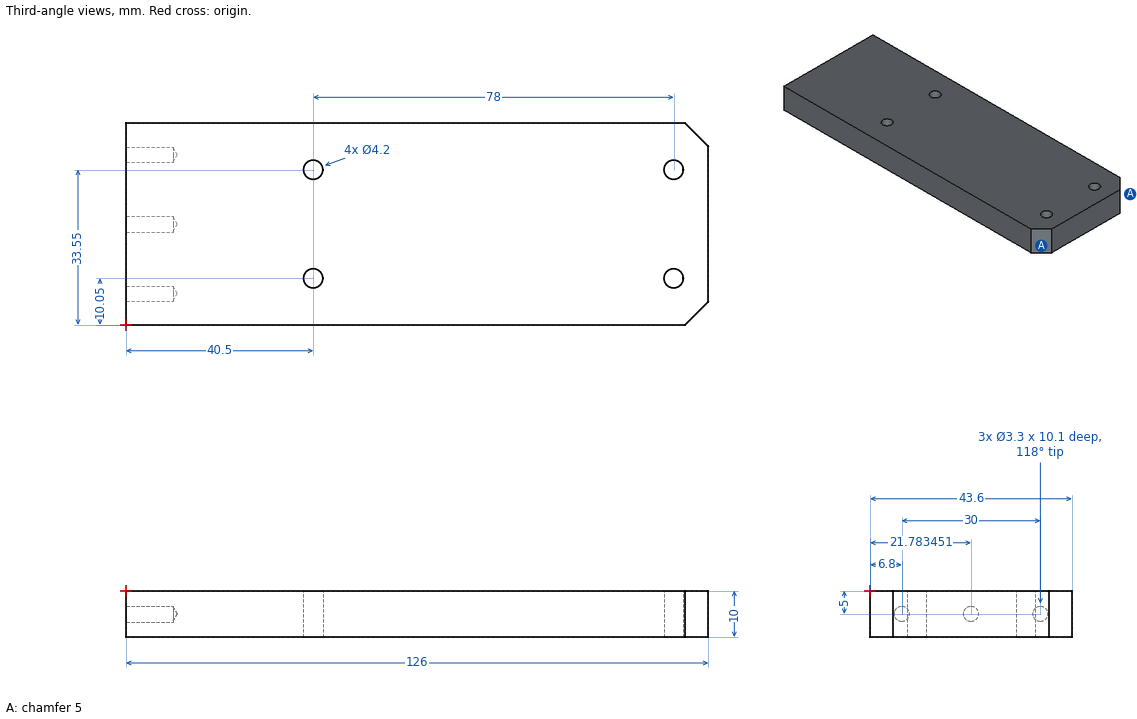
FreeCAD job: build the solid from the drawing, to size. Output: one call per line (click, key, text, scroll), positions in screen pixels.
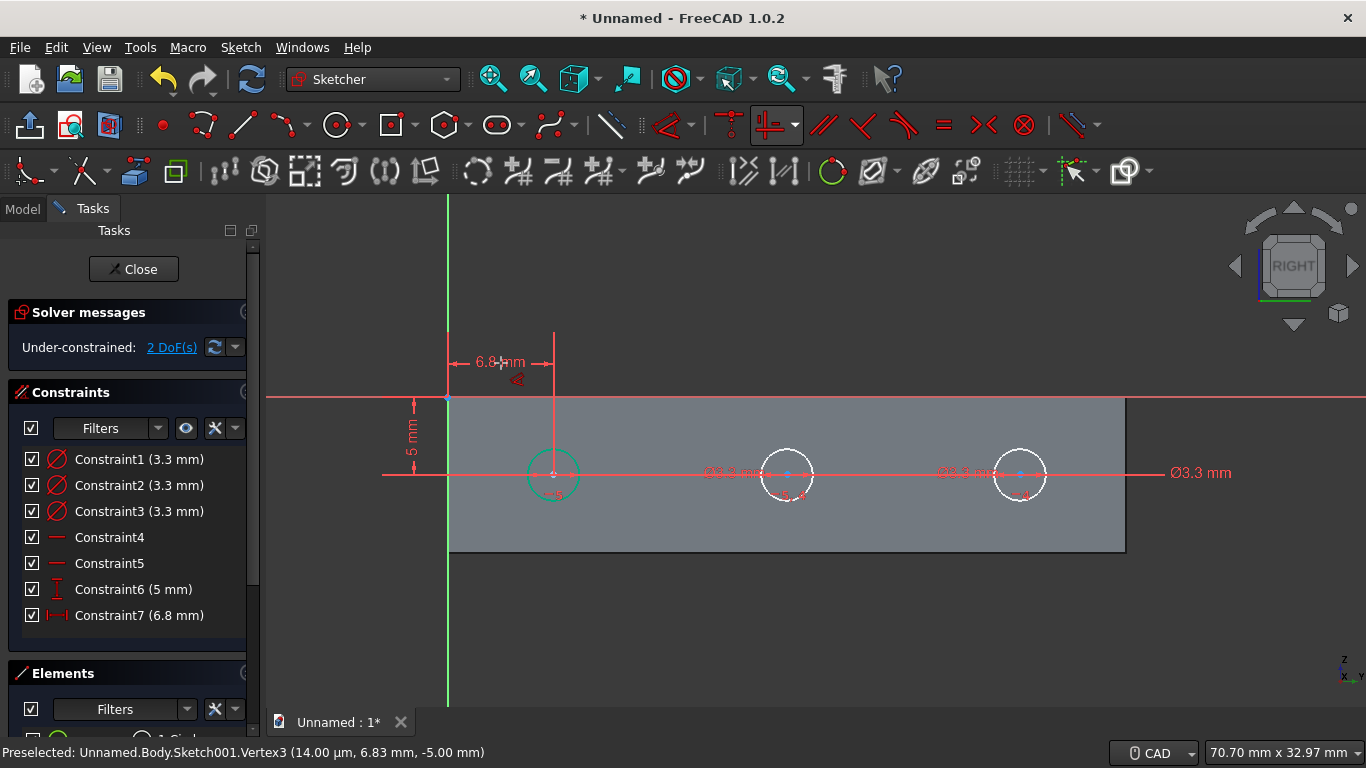
click(1020, 475)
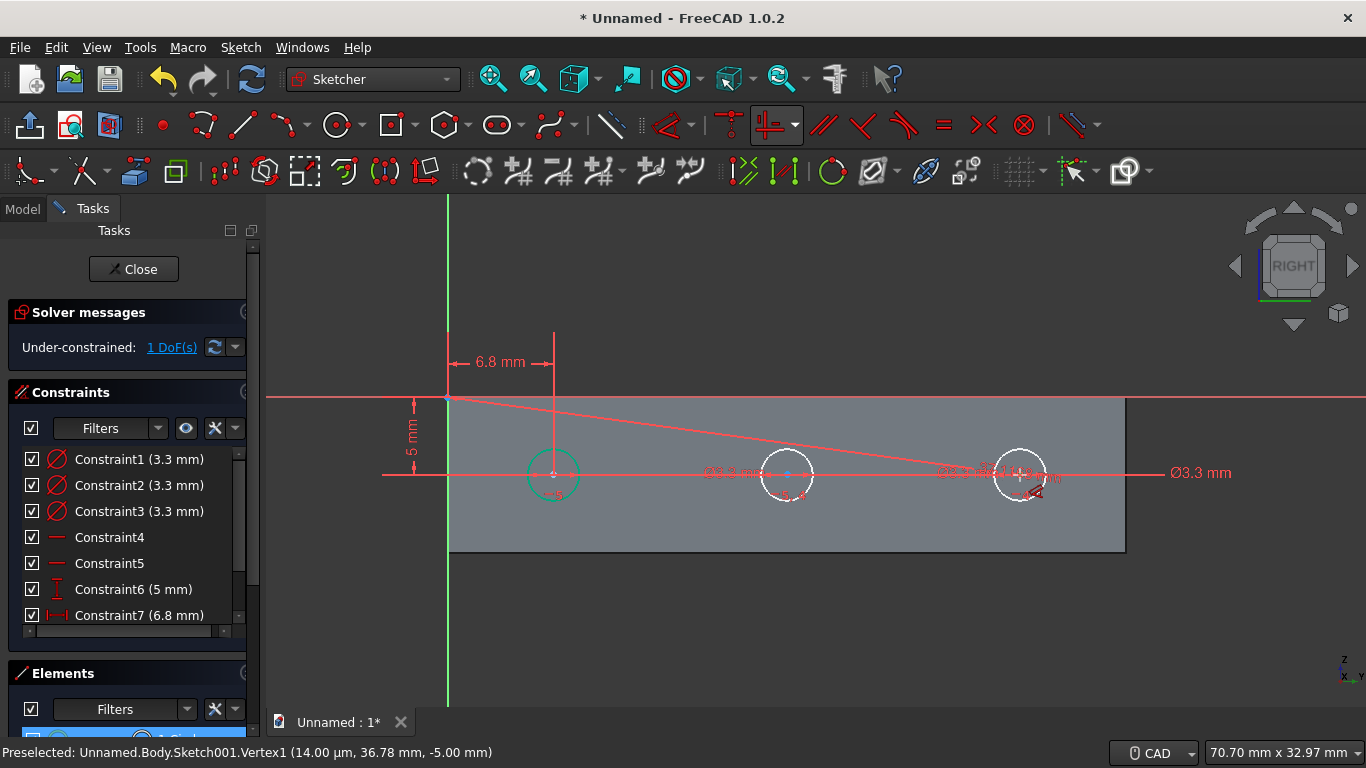
click(554, 475)
click(680, 509)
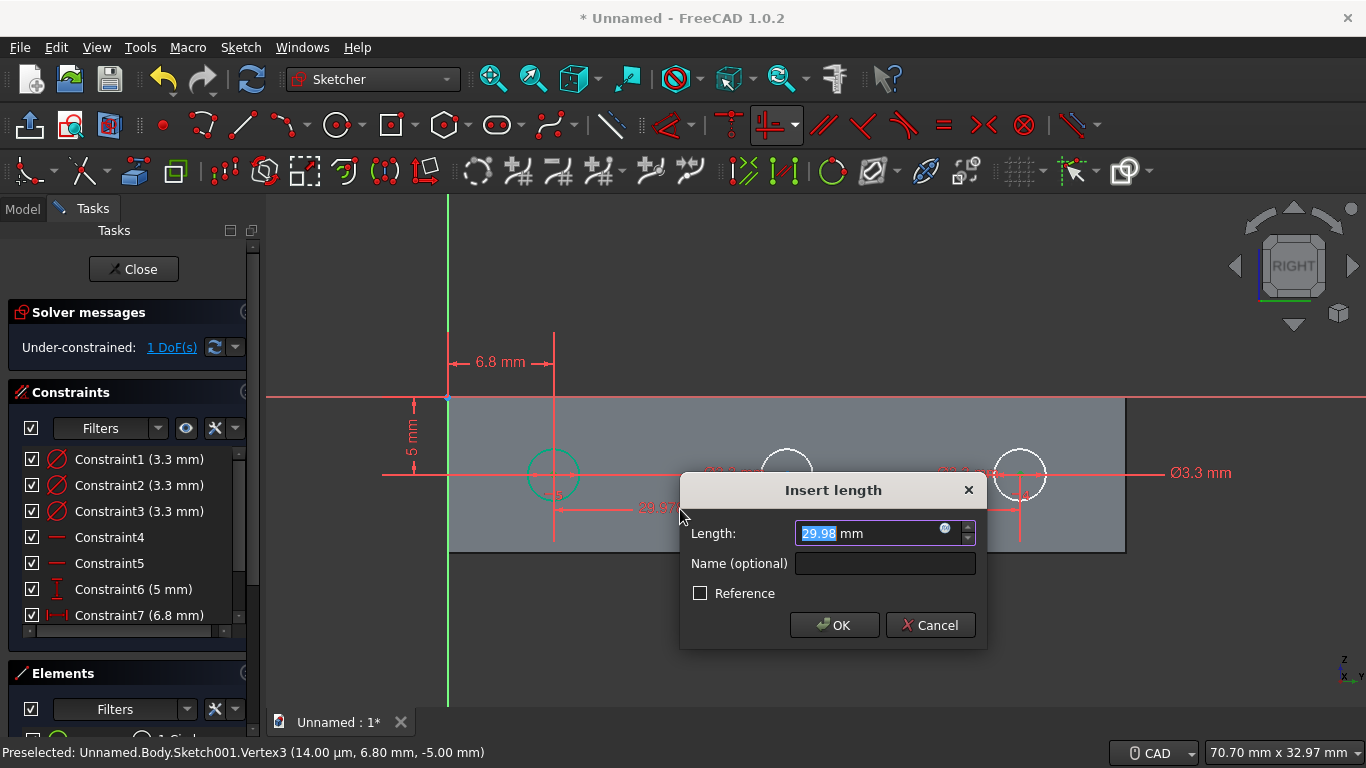
text(30)
key(Return)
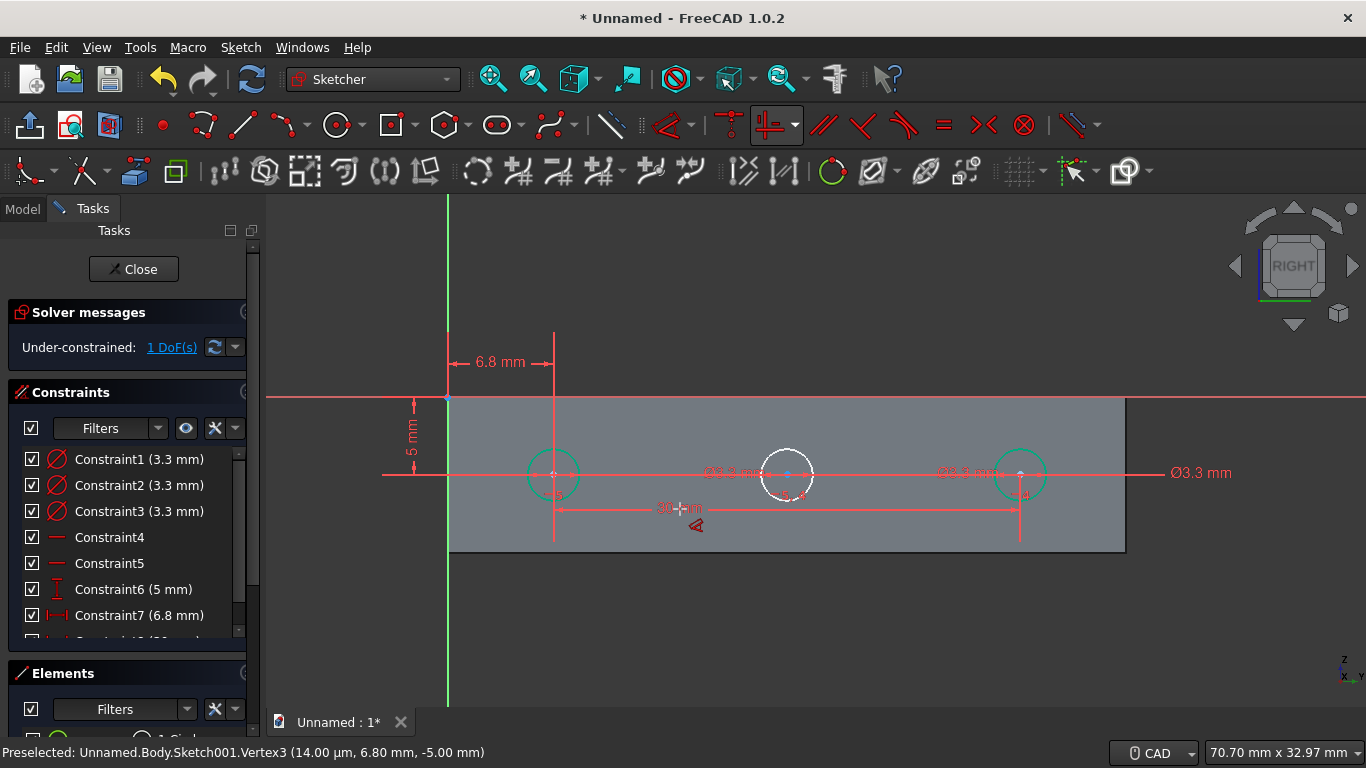
click(787, 475)
click(617, 363)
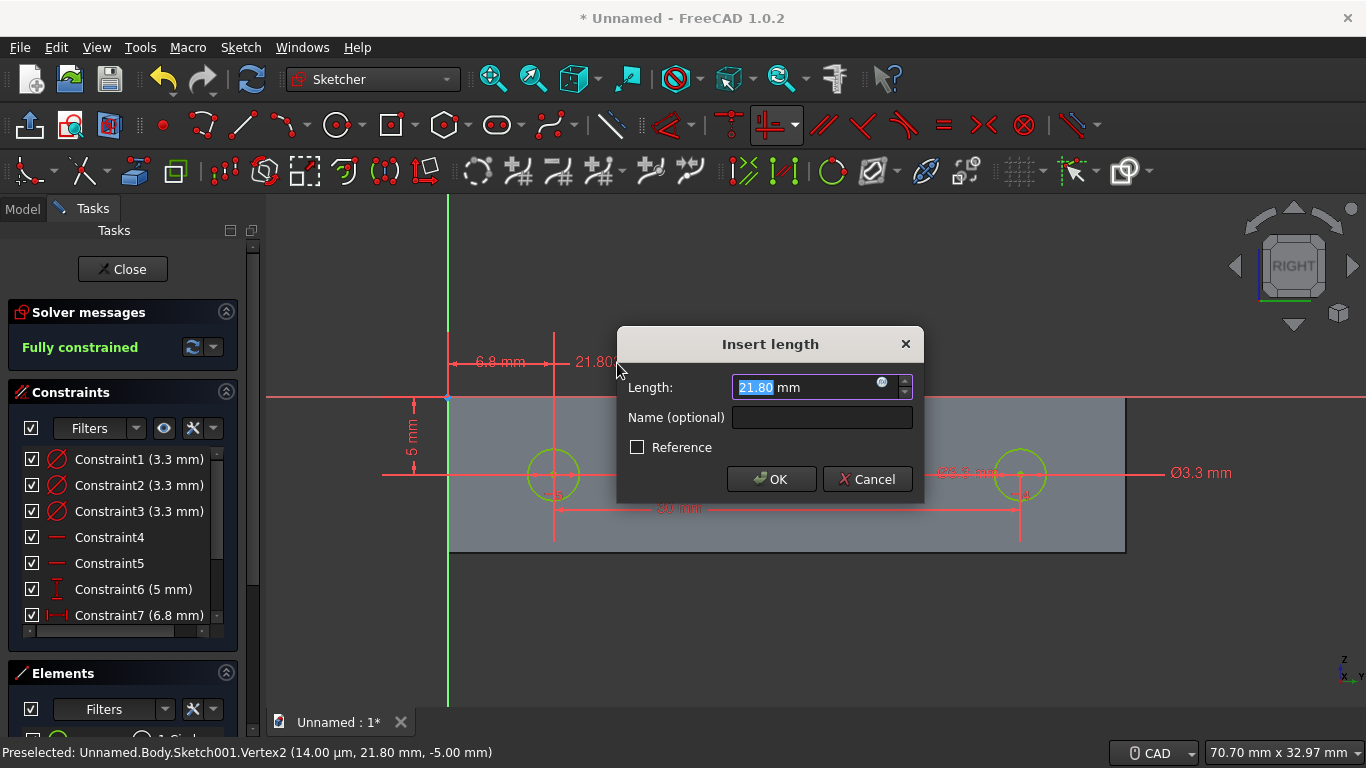
text(21.783451)
key(Return)
key(Escape)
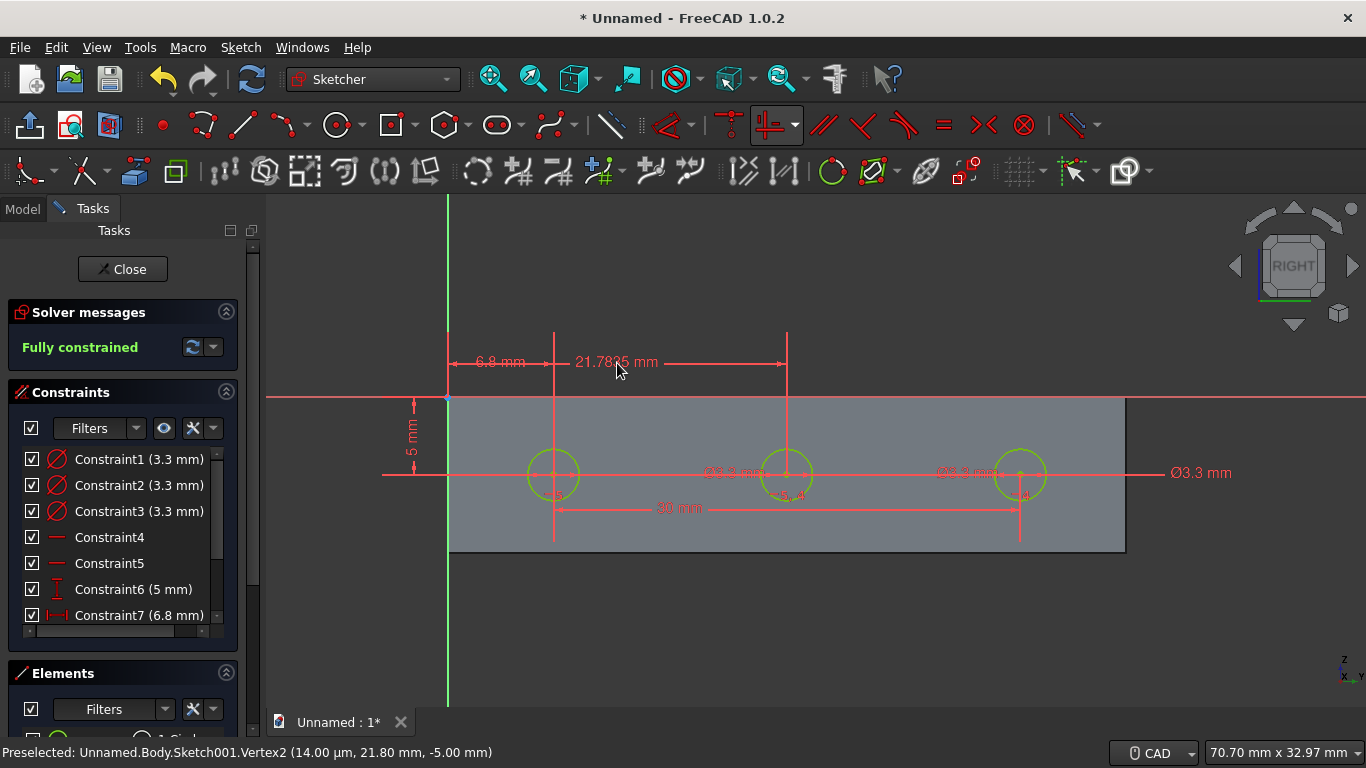
click(123, 269)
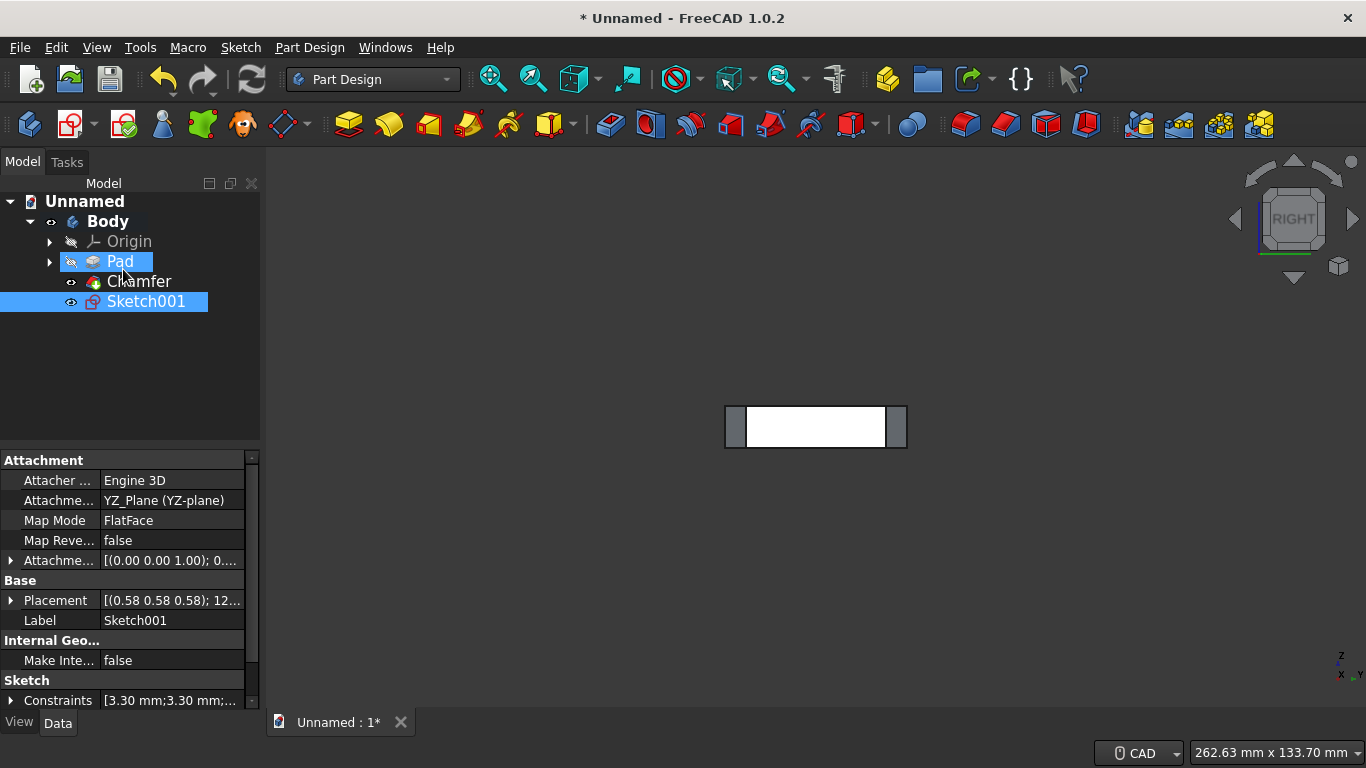
click(652, 124)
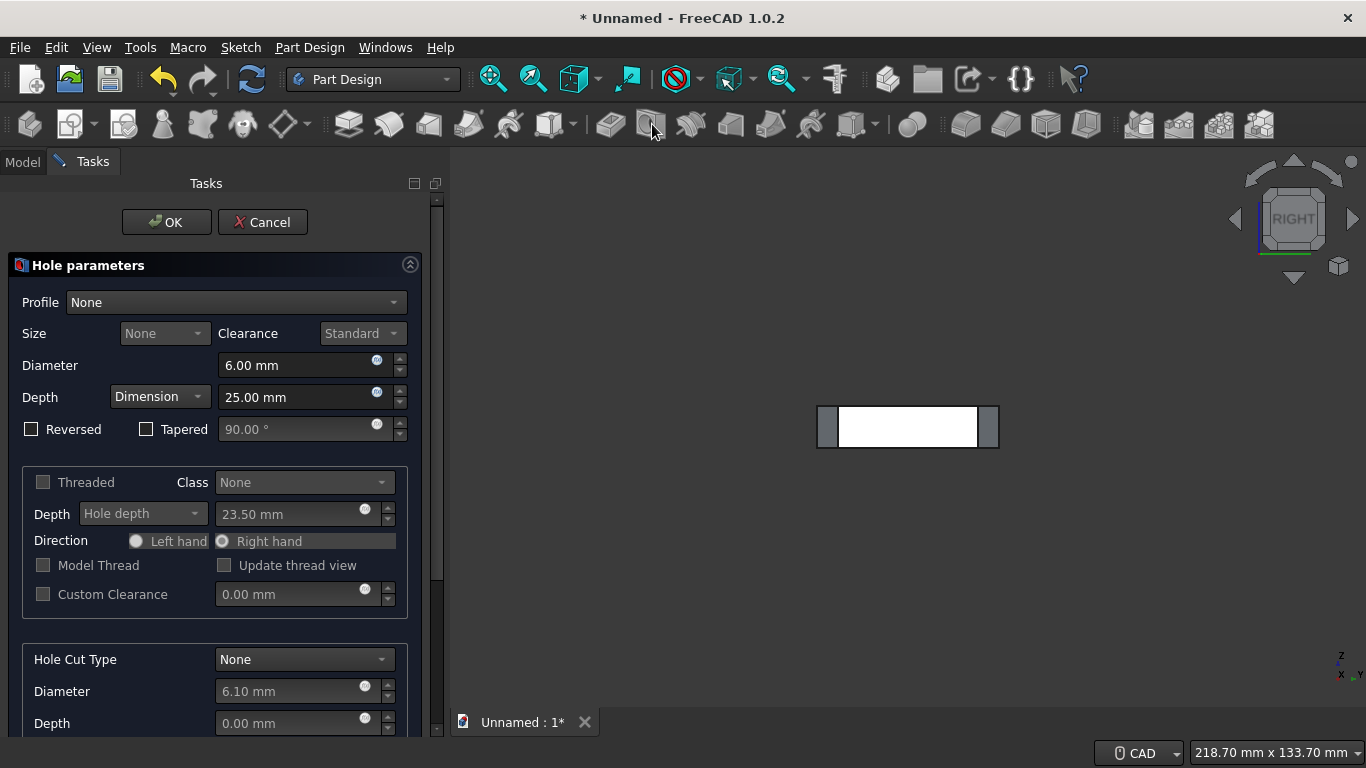
triple_click(305, 365)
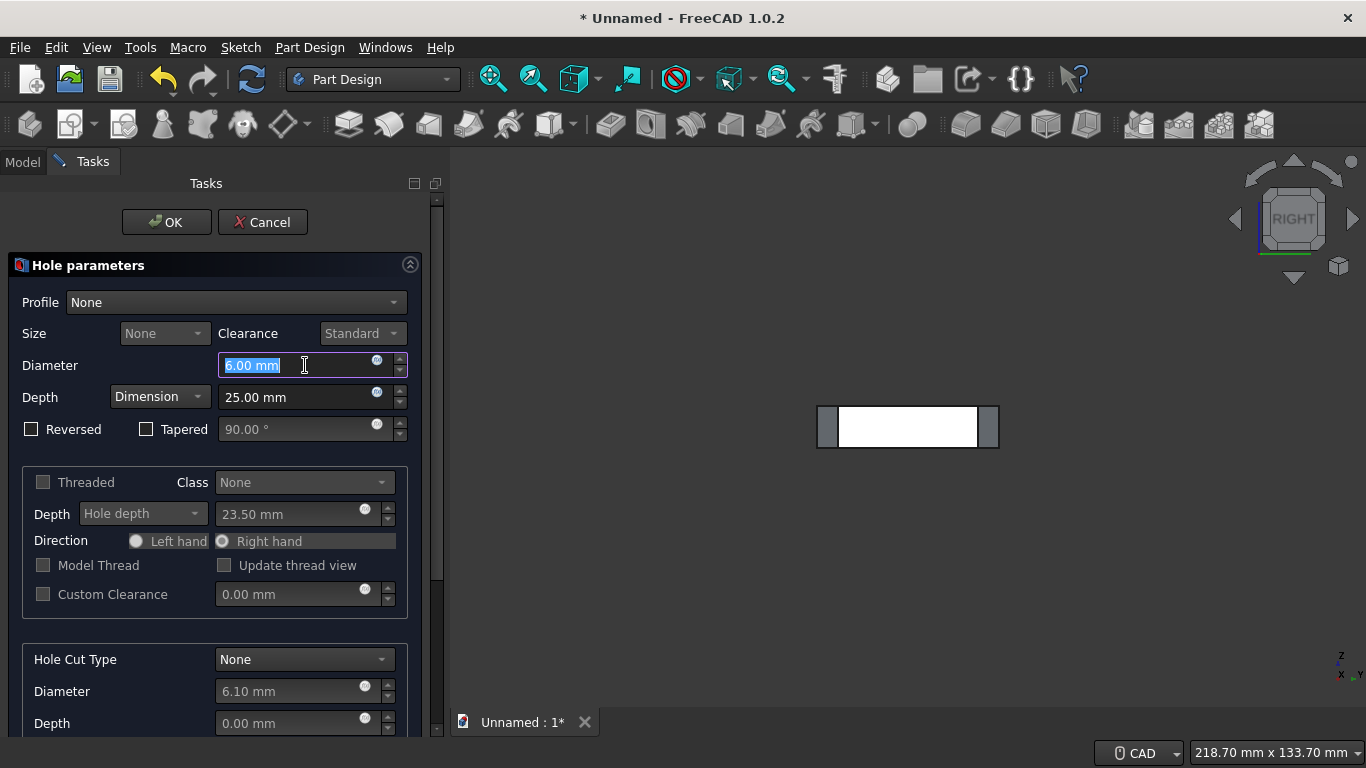
text(3.3)
key(Tab)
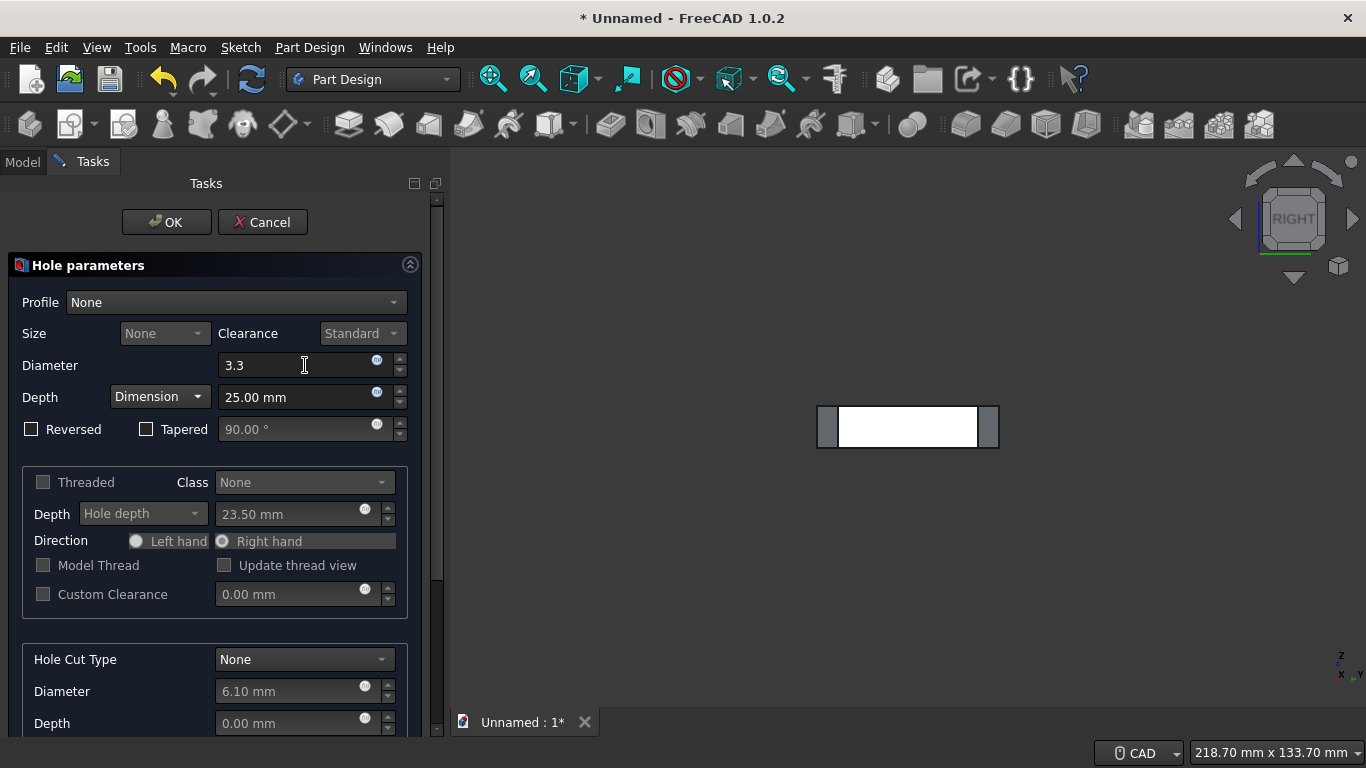
triple_click(305, 397)